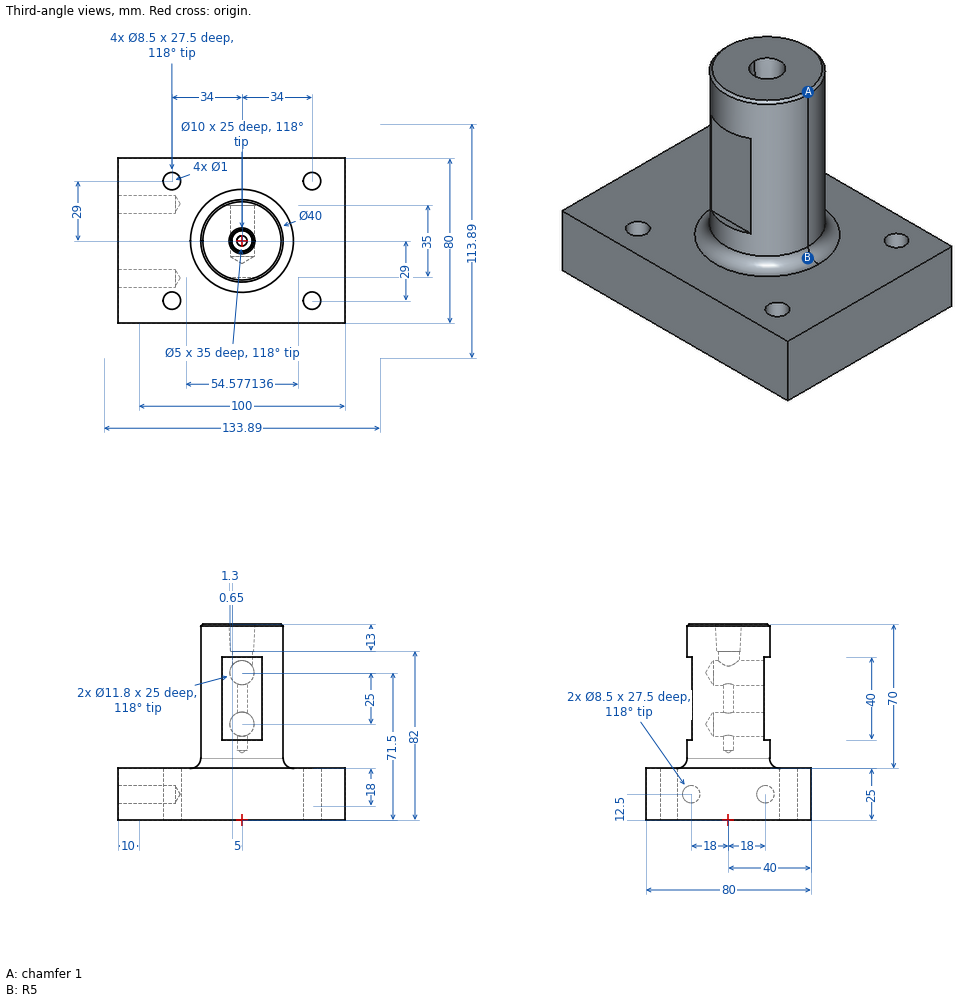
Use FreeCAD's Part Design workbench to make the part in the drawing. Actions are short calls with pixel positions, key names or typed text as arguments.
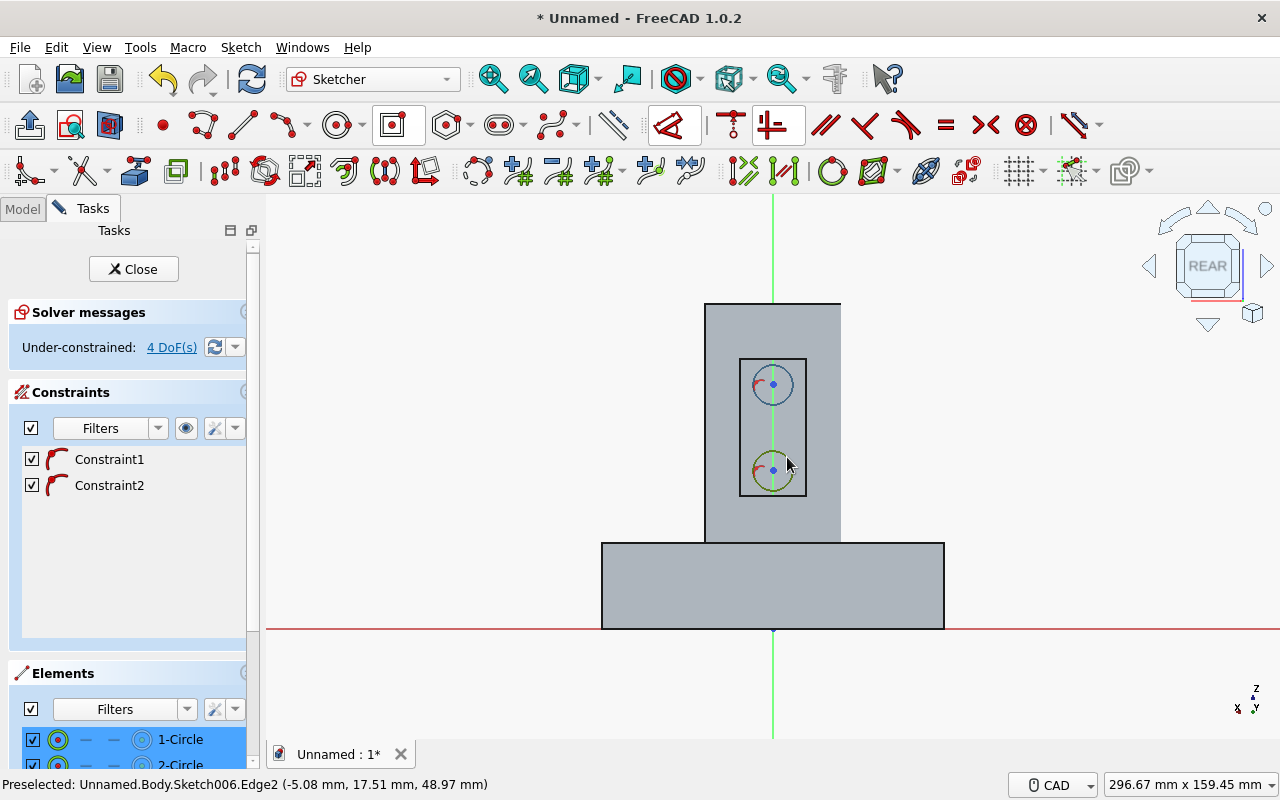
click(946, 126)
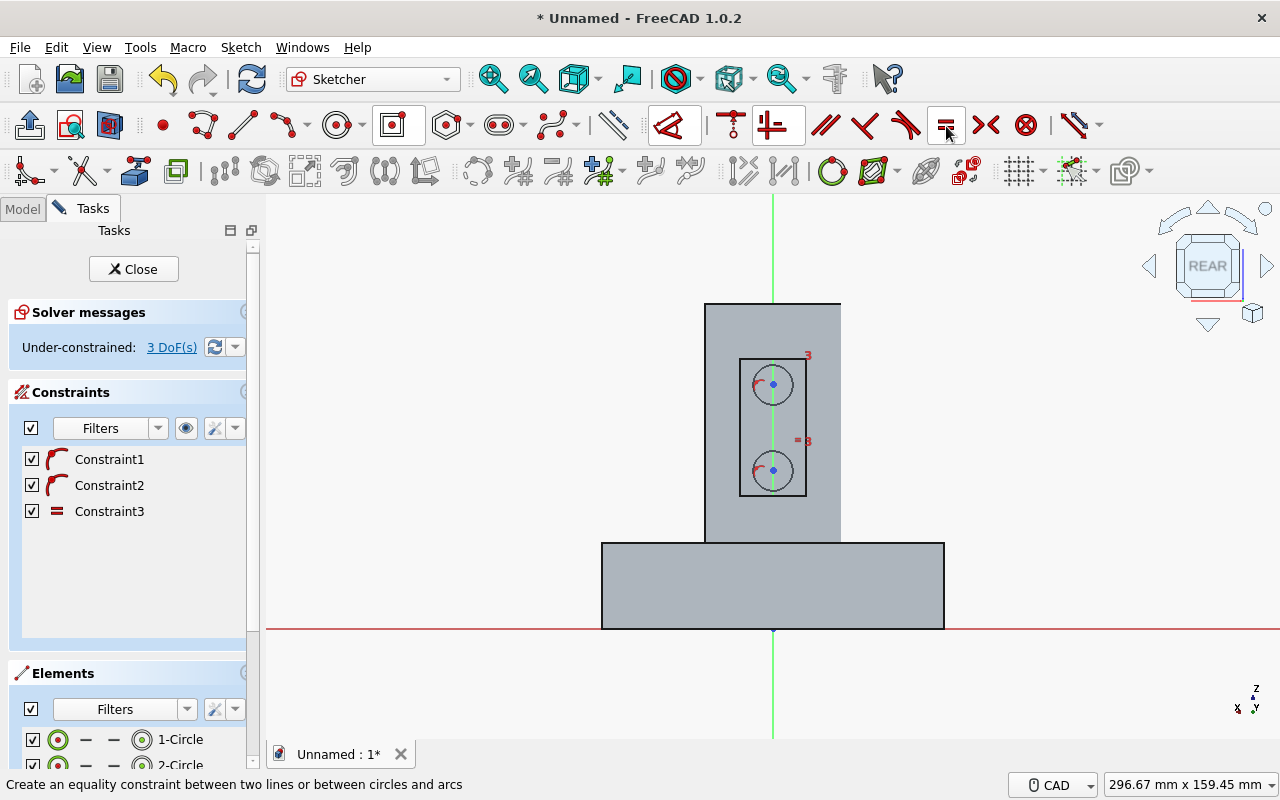
click(787, 371)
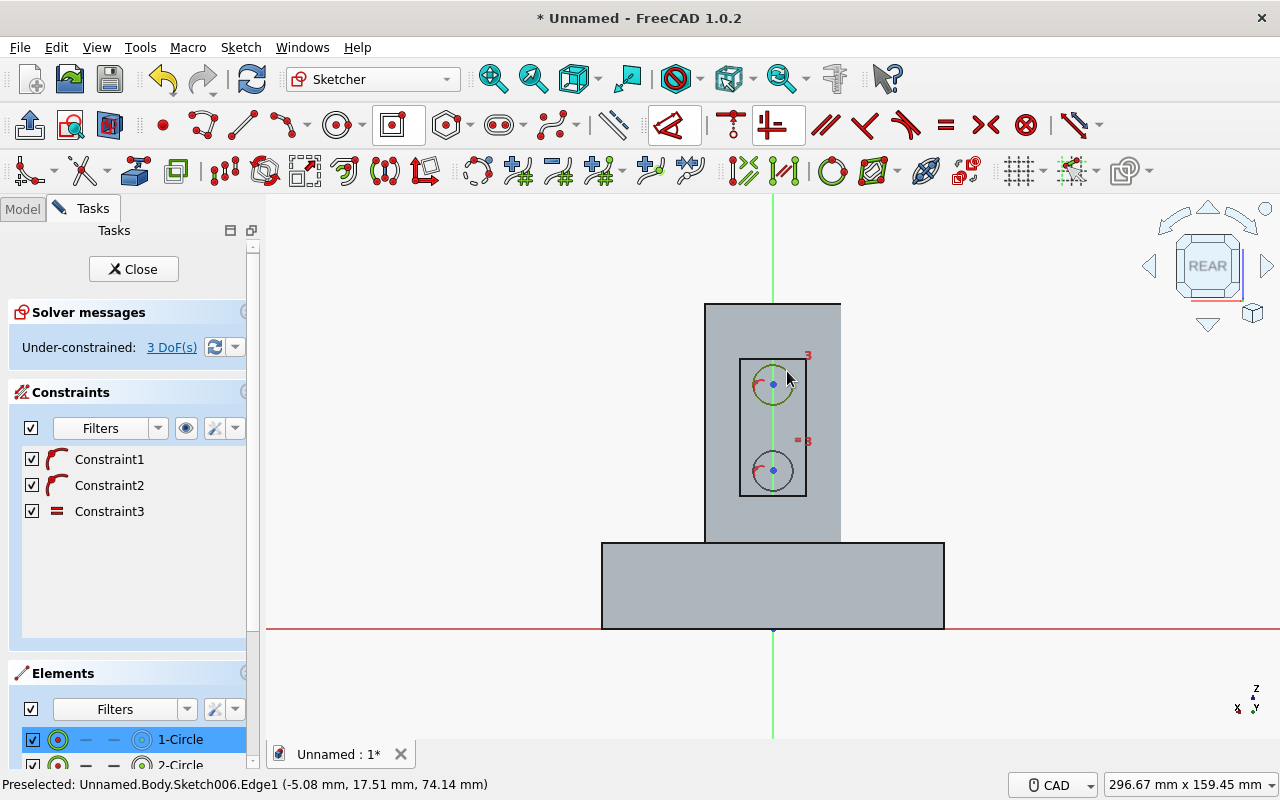
key(k)
key(o)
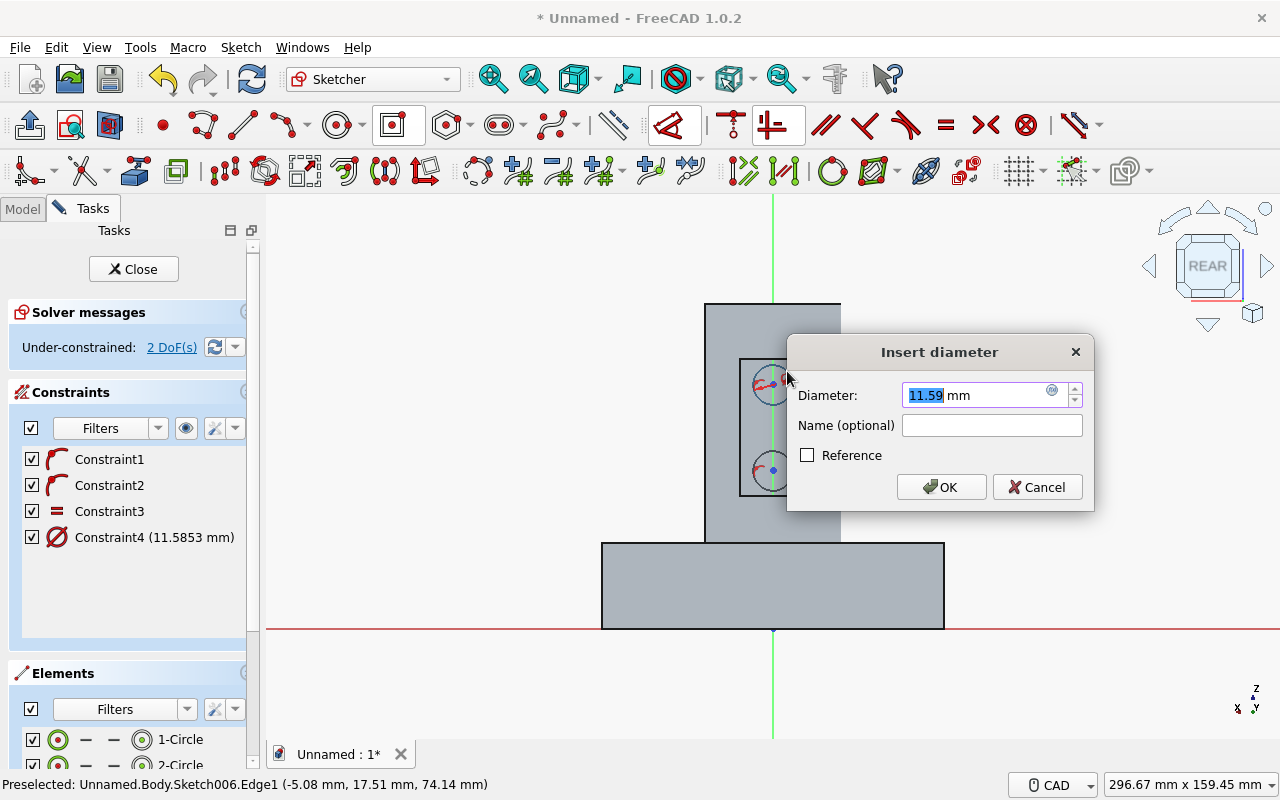
text(11.8)
key(Return)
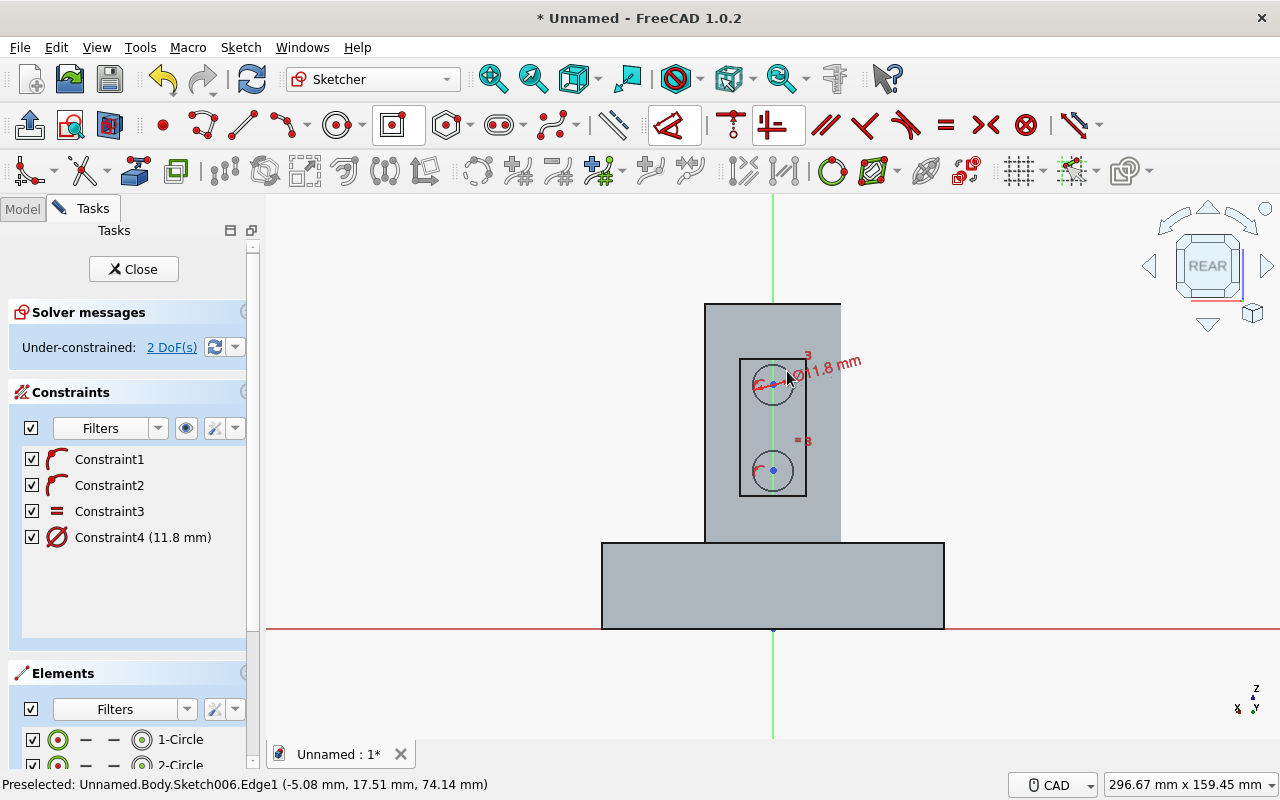
click(773, 385)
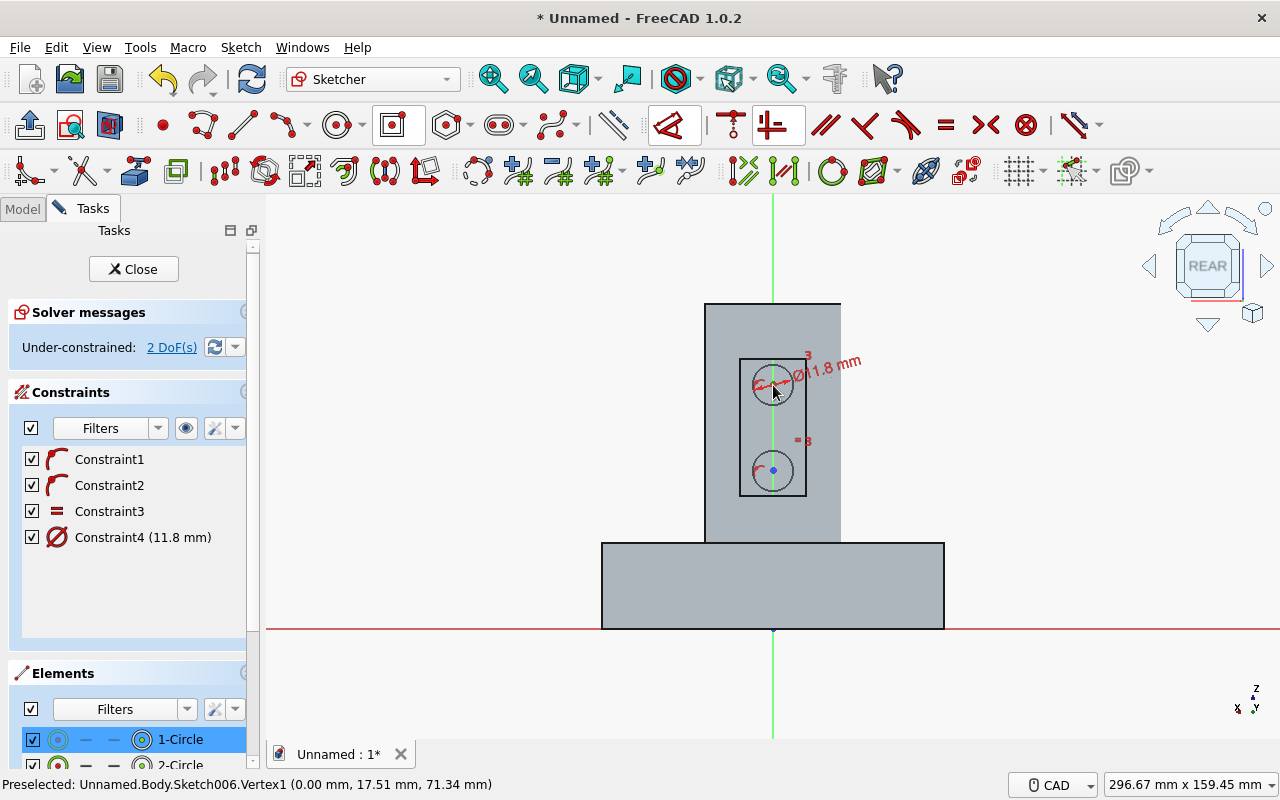
click(773, 471)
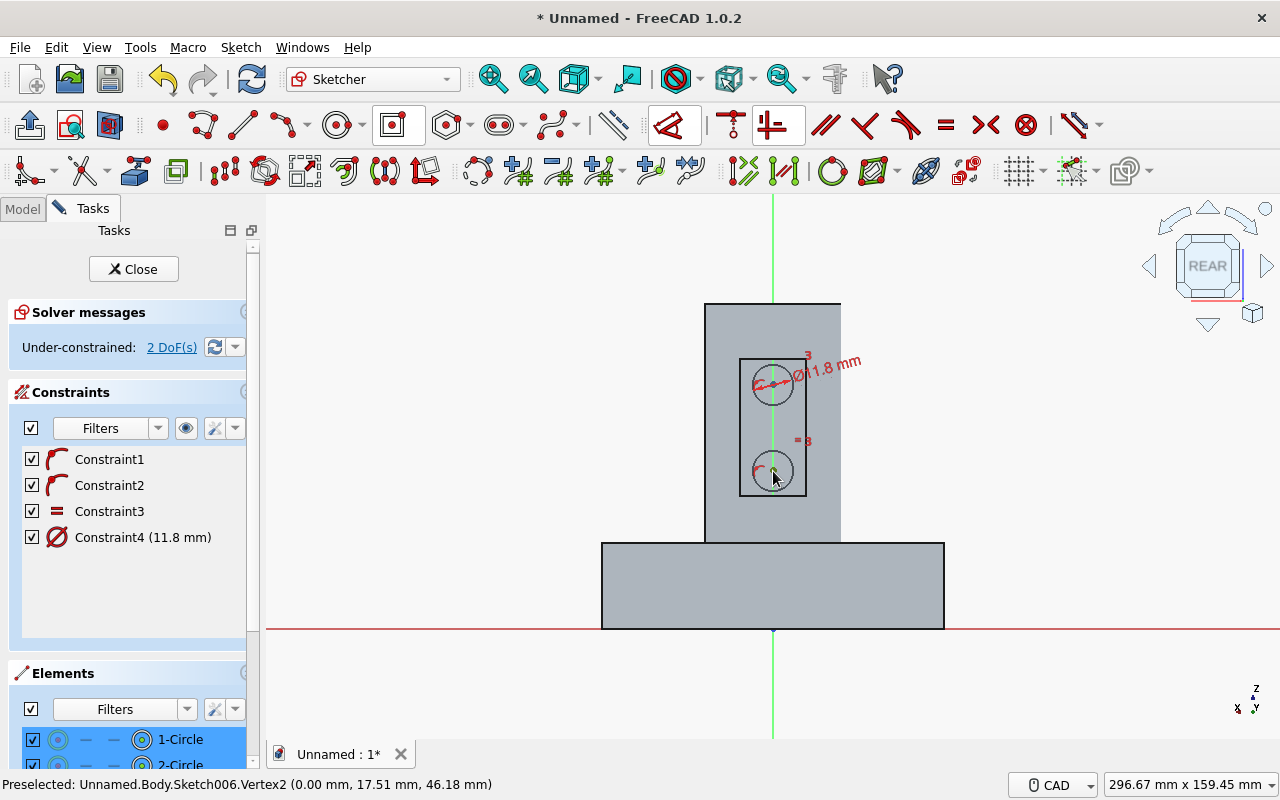
key(i)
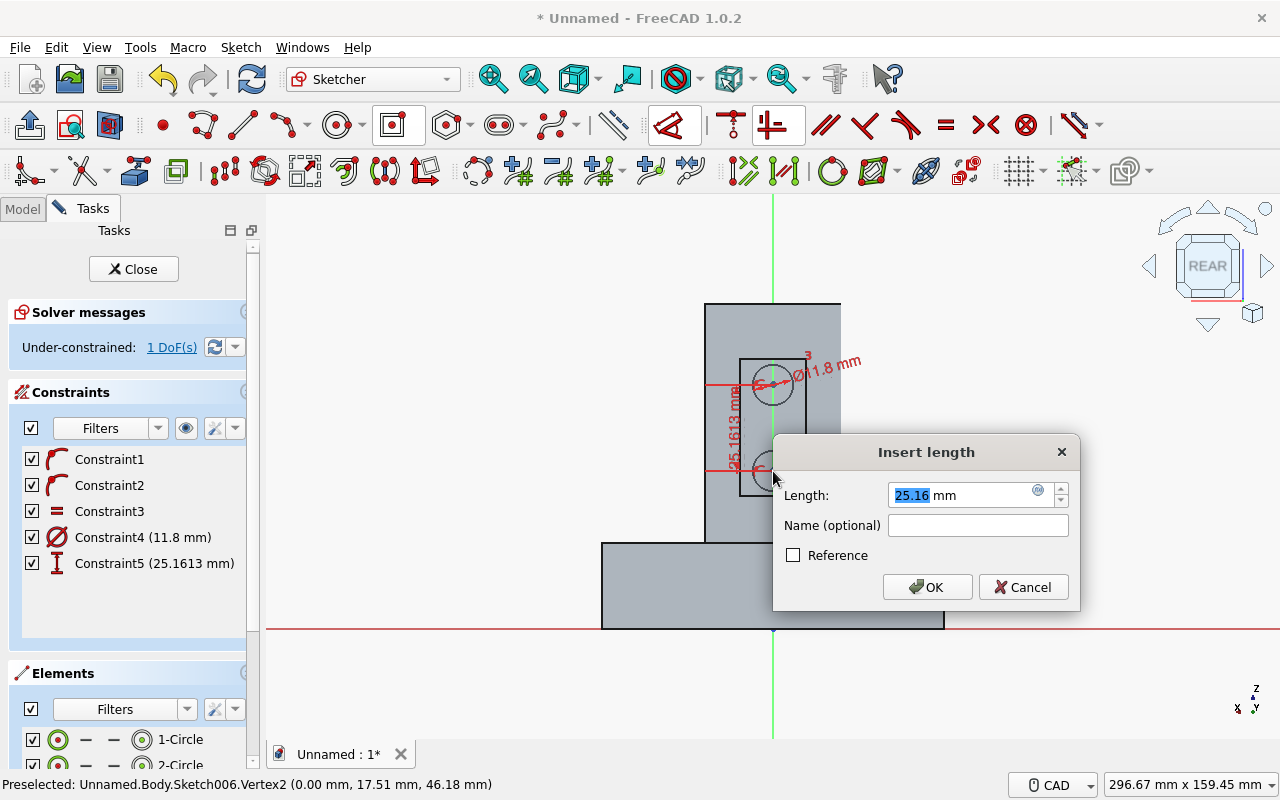
text(25)
key(Return)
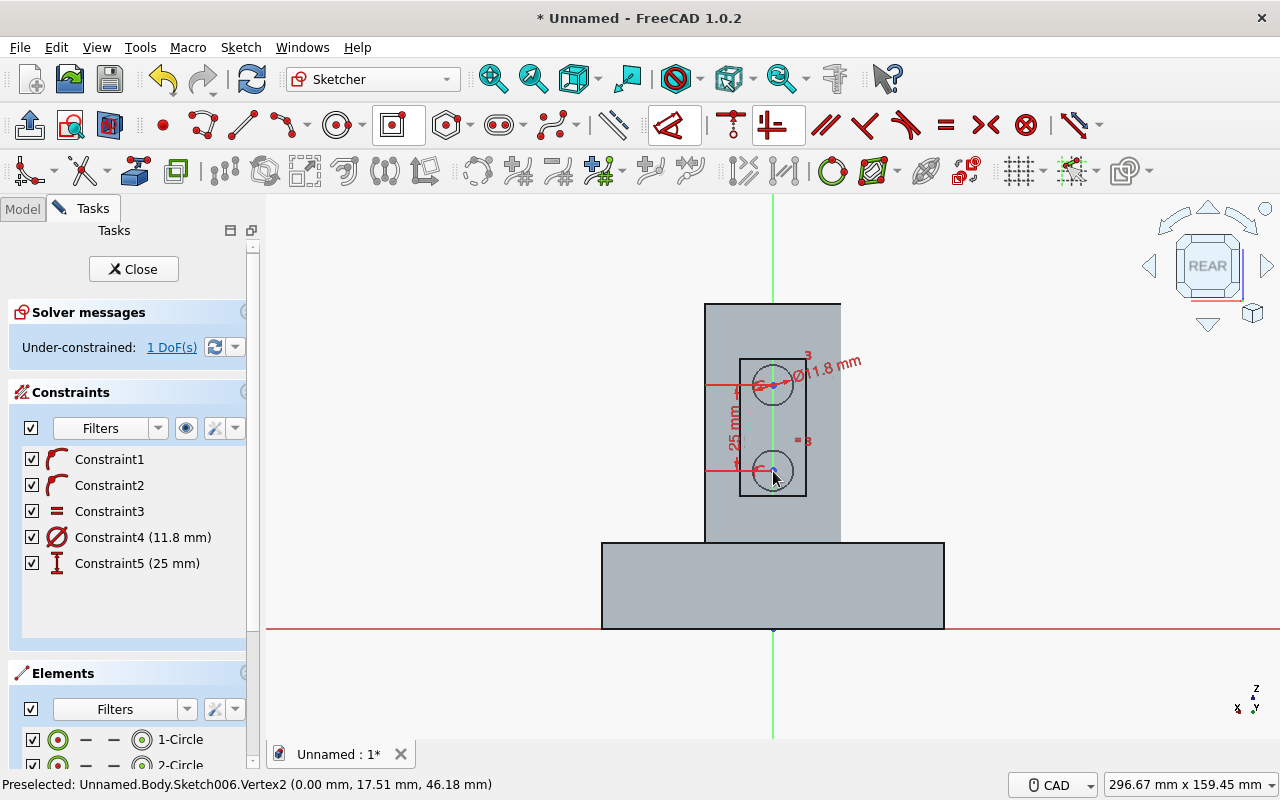
click(773, 385)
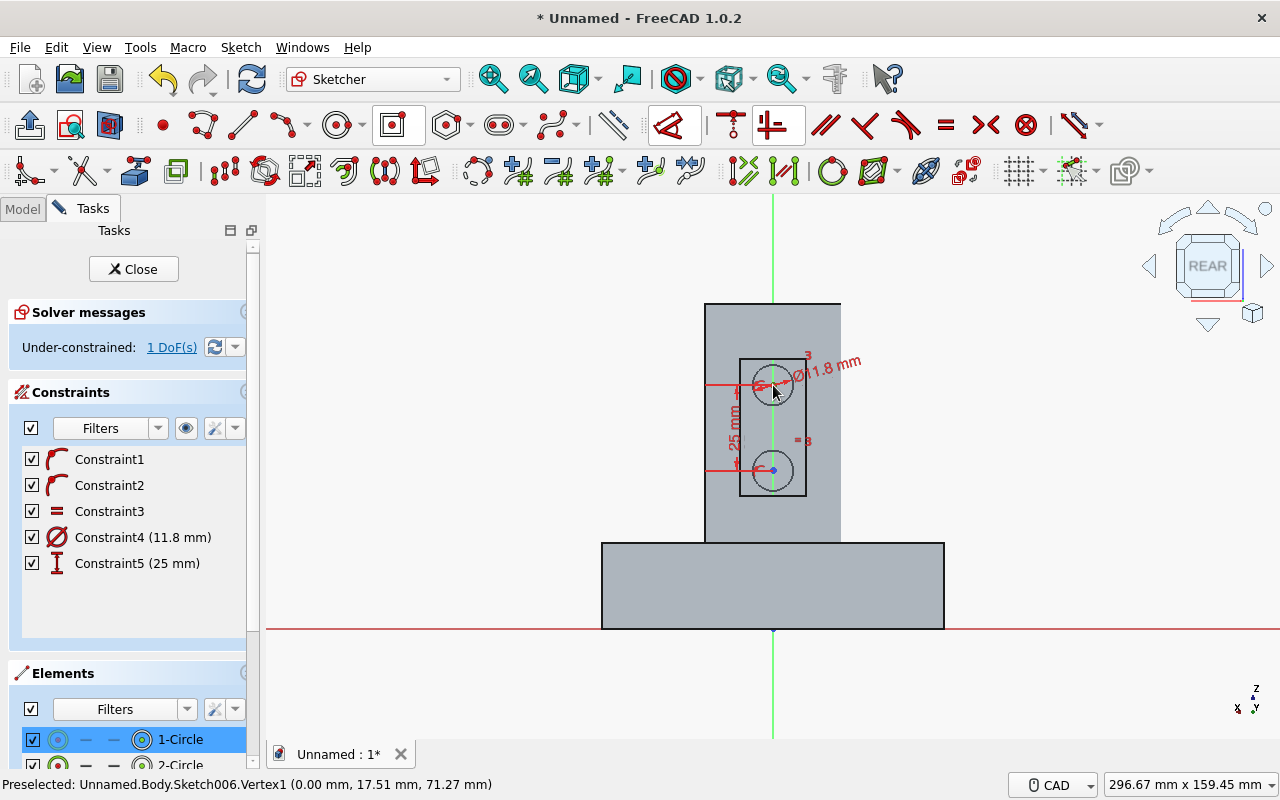
key(i)